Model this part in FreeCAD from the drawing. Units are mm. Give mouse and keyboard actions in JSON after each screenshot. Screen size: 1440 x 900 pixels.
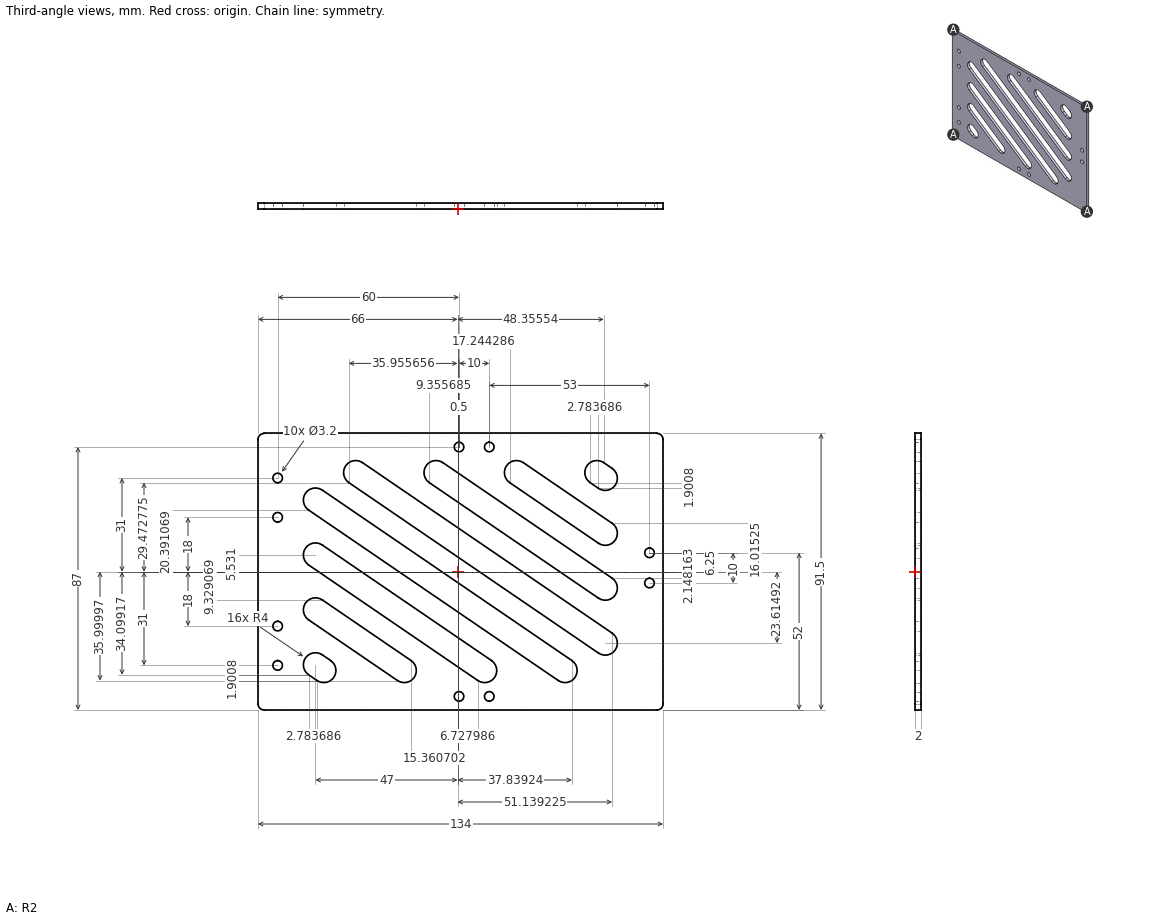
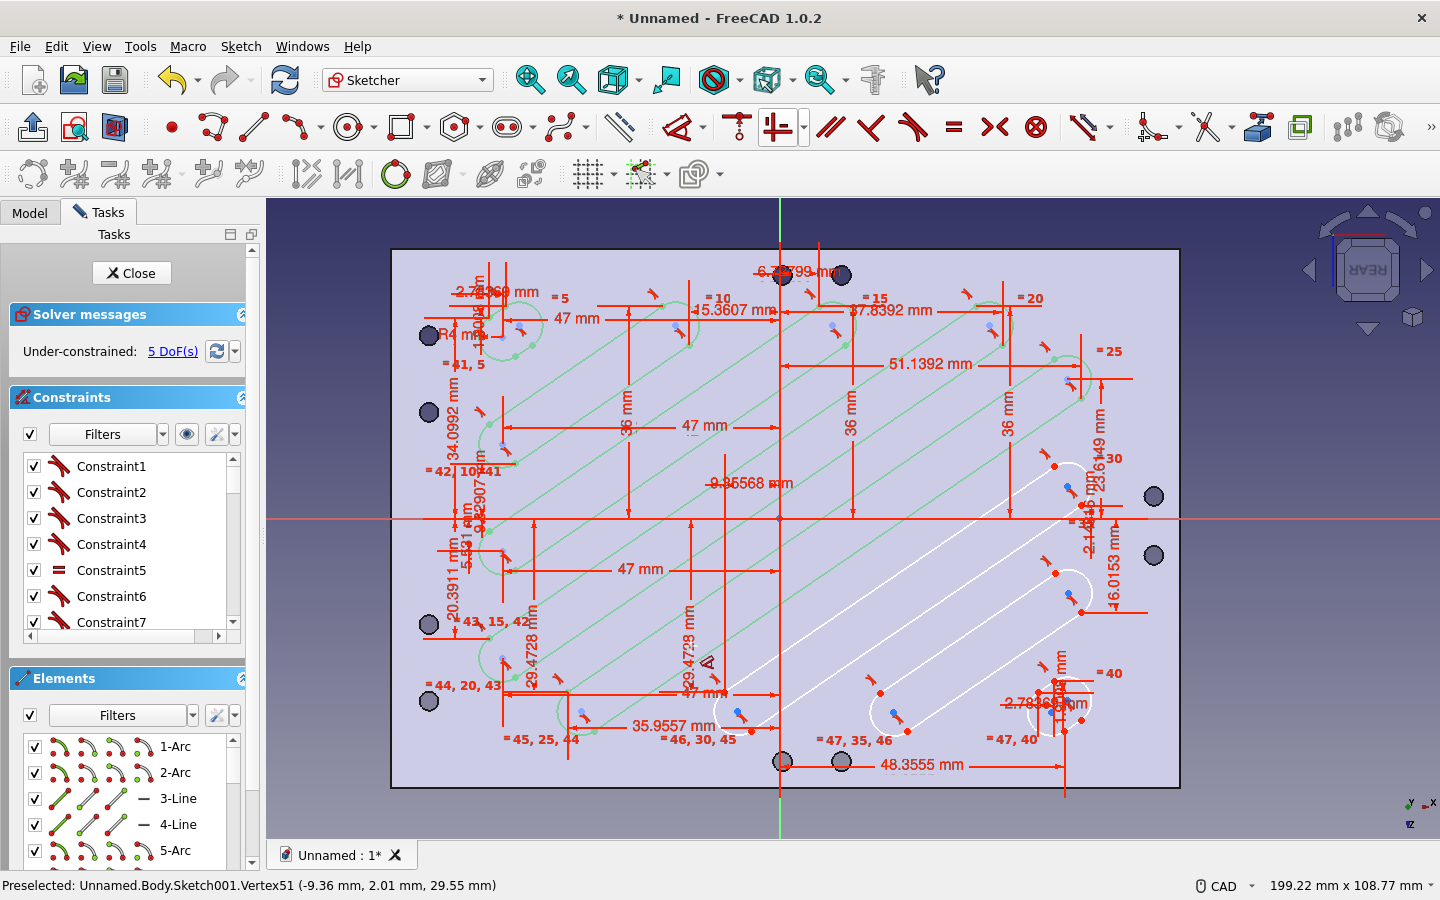
{"action": "left_click", "coordinate": [1081, 506]}
{"action": "left_click", "coordinate": [930, 472]}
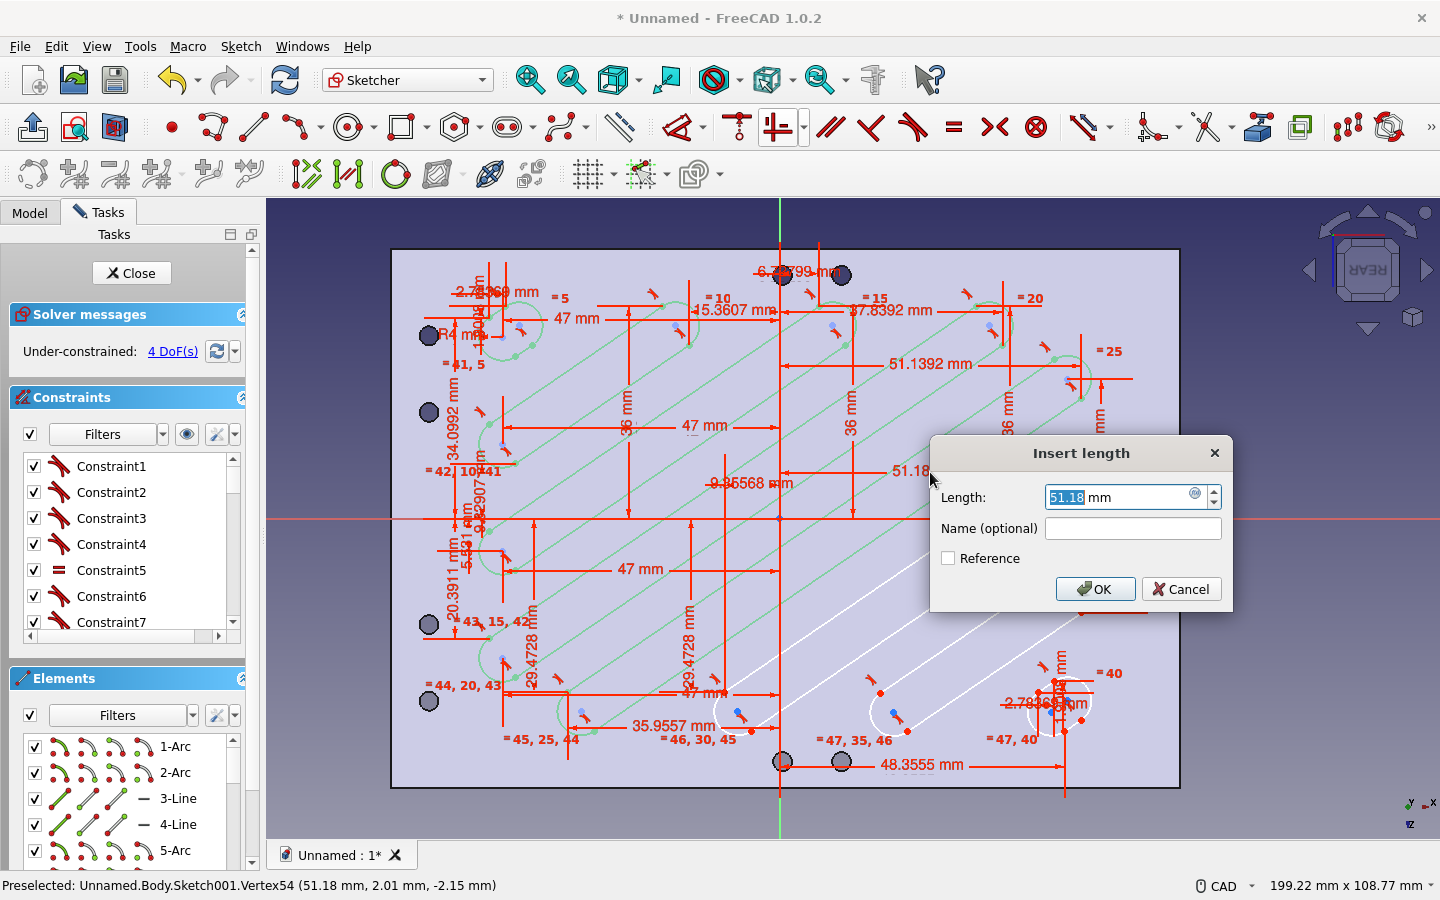
{"action": "type", "text": "51.139225"}
{"action": "key", "text": "Return"}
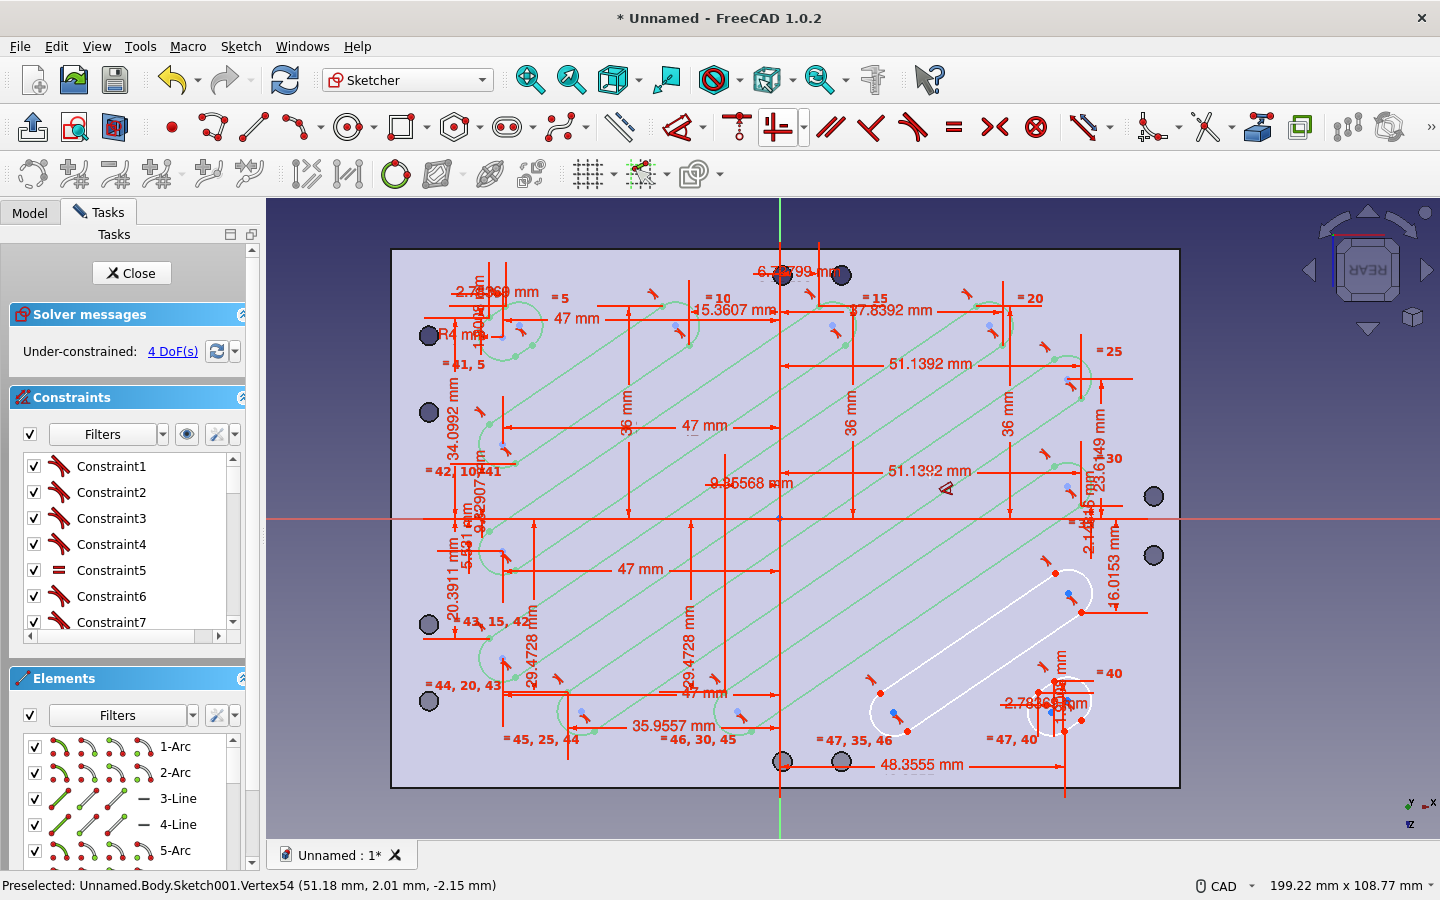
{"action": "left_click", "coordinate": [881, 693]}
{"action": "left_click", "coordinate": [830, 727]}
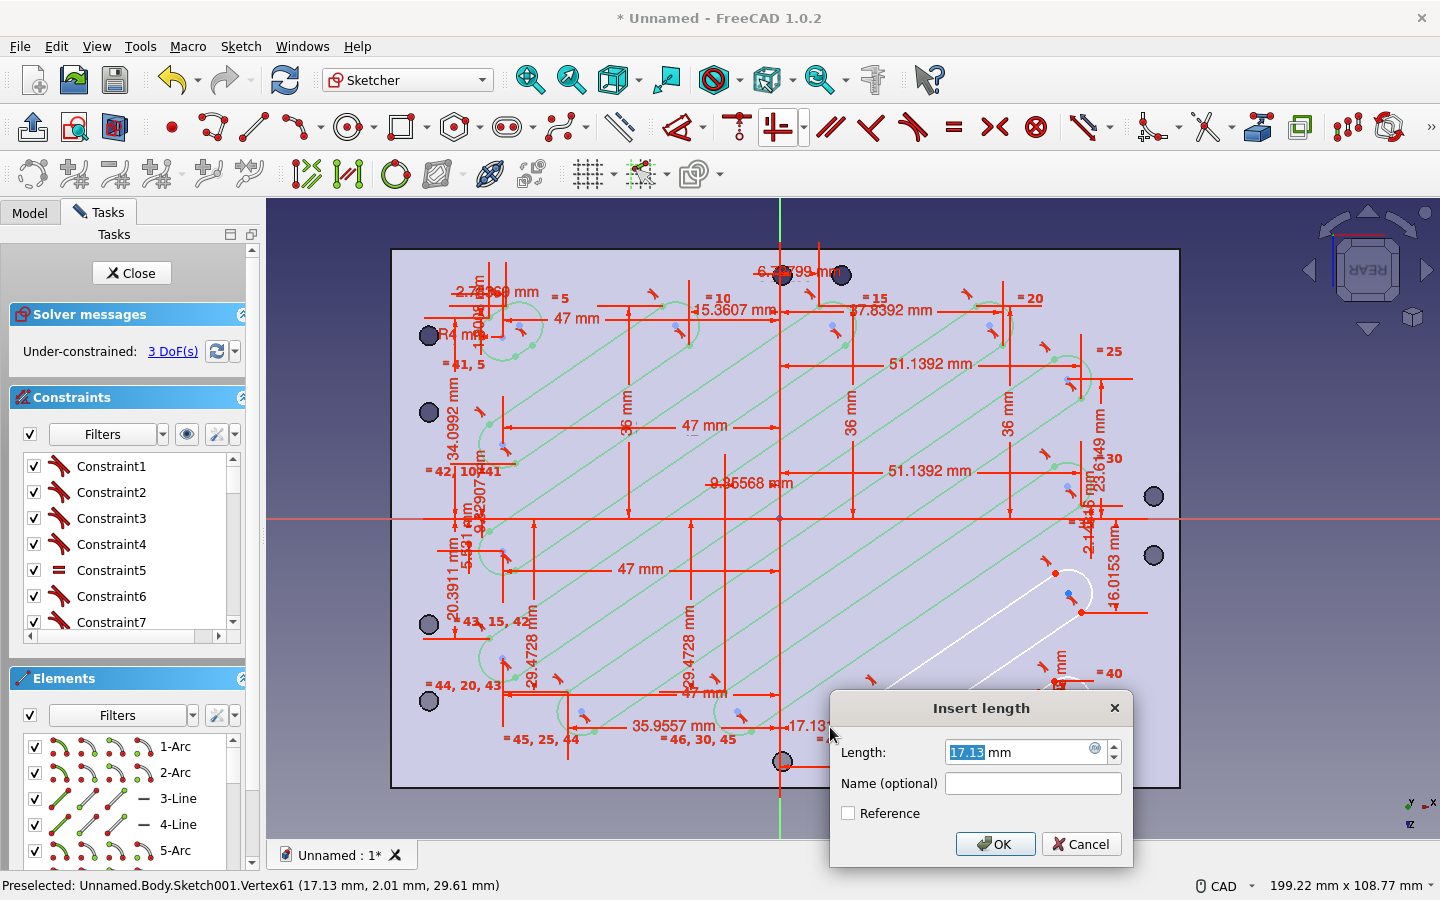
{"action": "type", "text": "17.244286"}
{"action": "key", "text": "Return"}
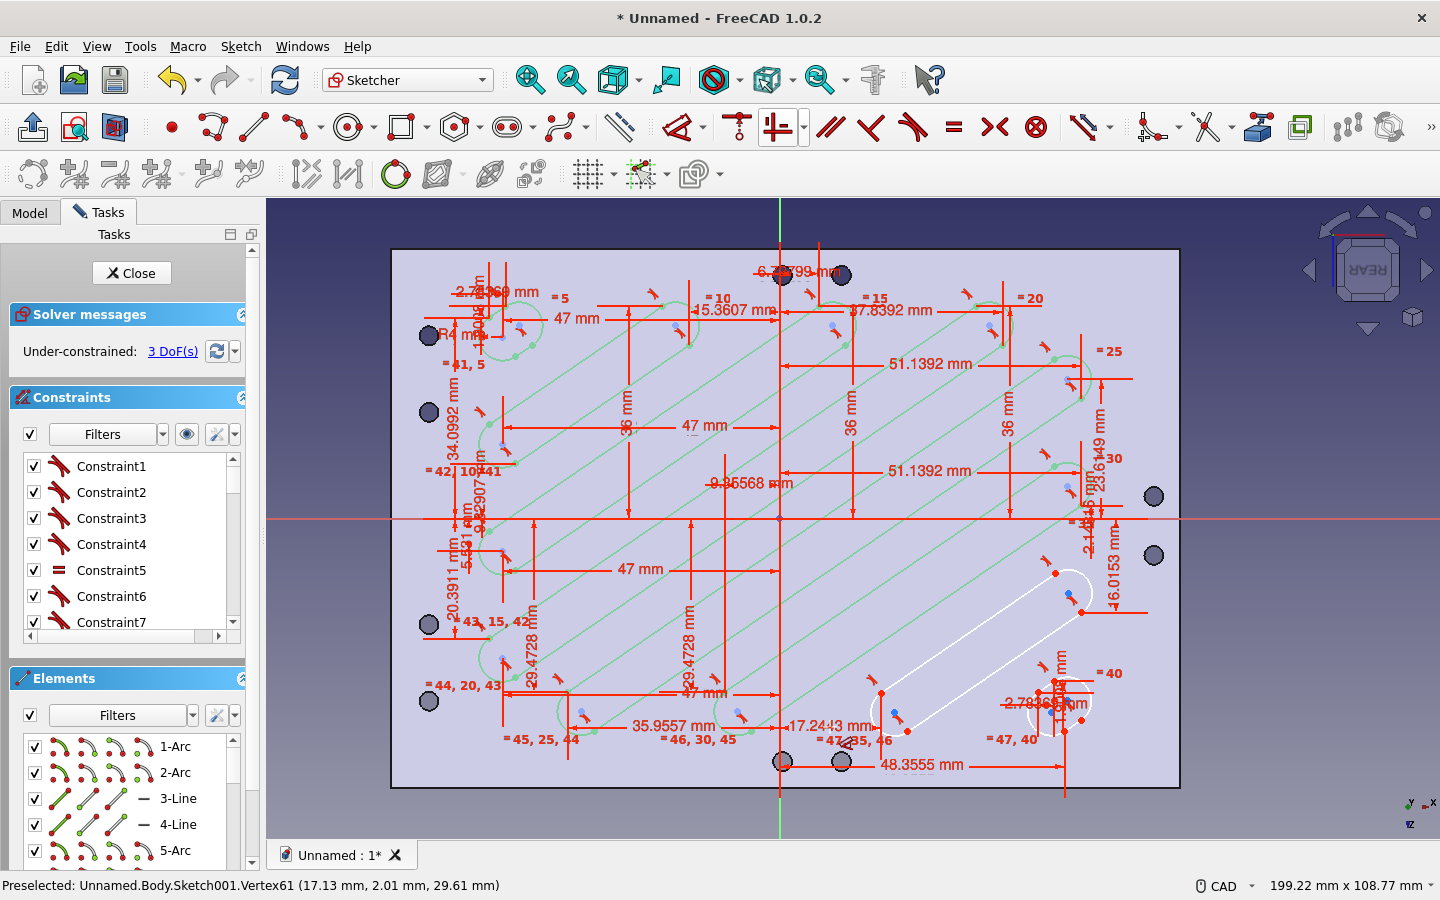
{"action": "left_click", "coordinate": [881, 693]}
{"action": "left_click", "coordinate": [915, 646]}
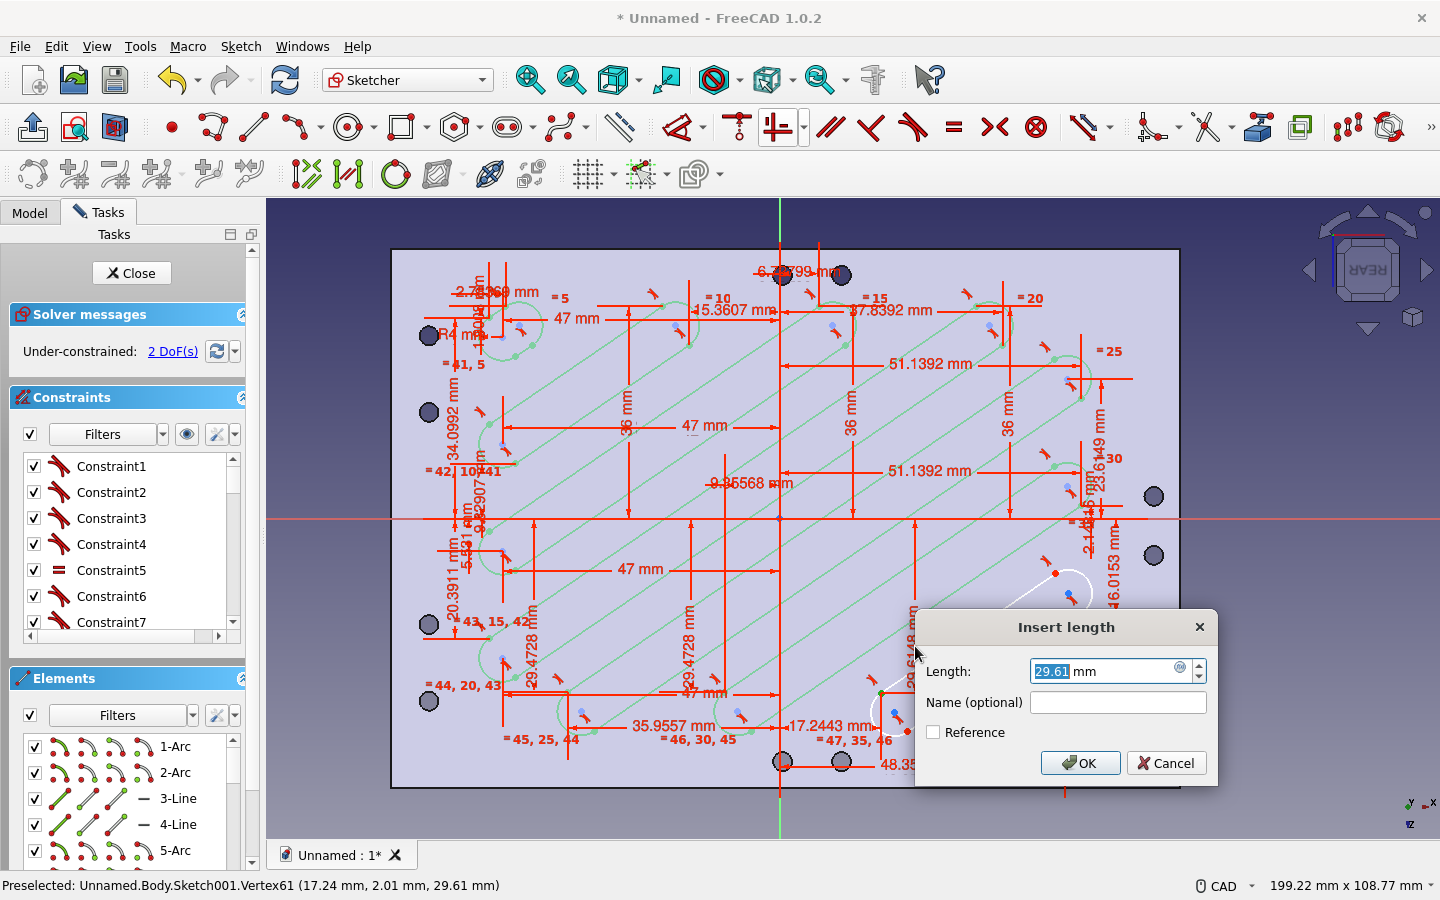
{"action": "type", "text": "29.472775"}
{"action": "key", "text": "Return"}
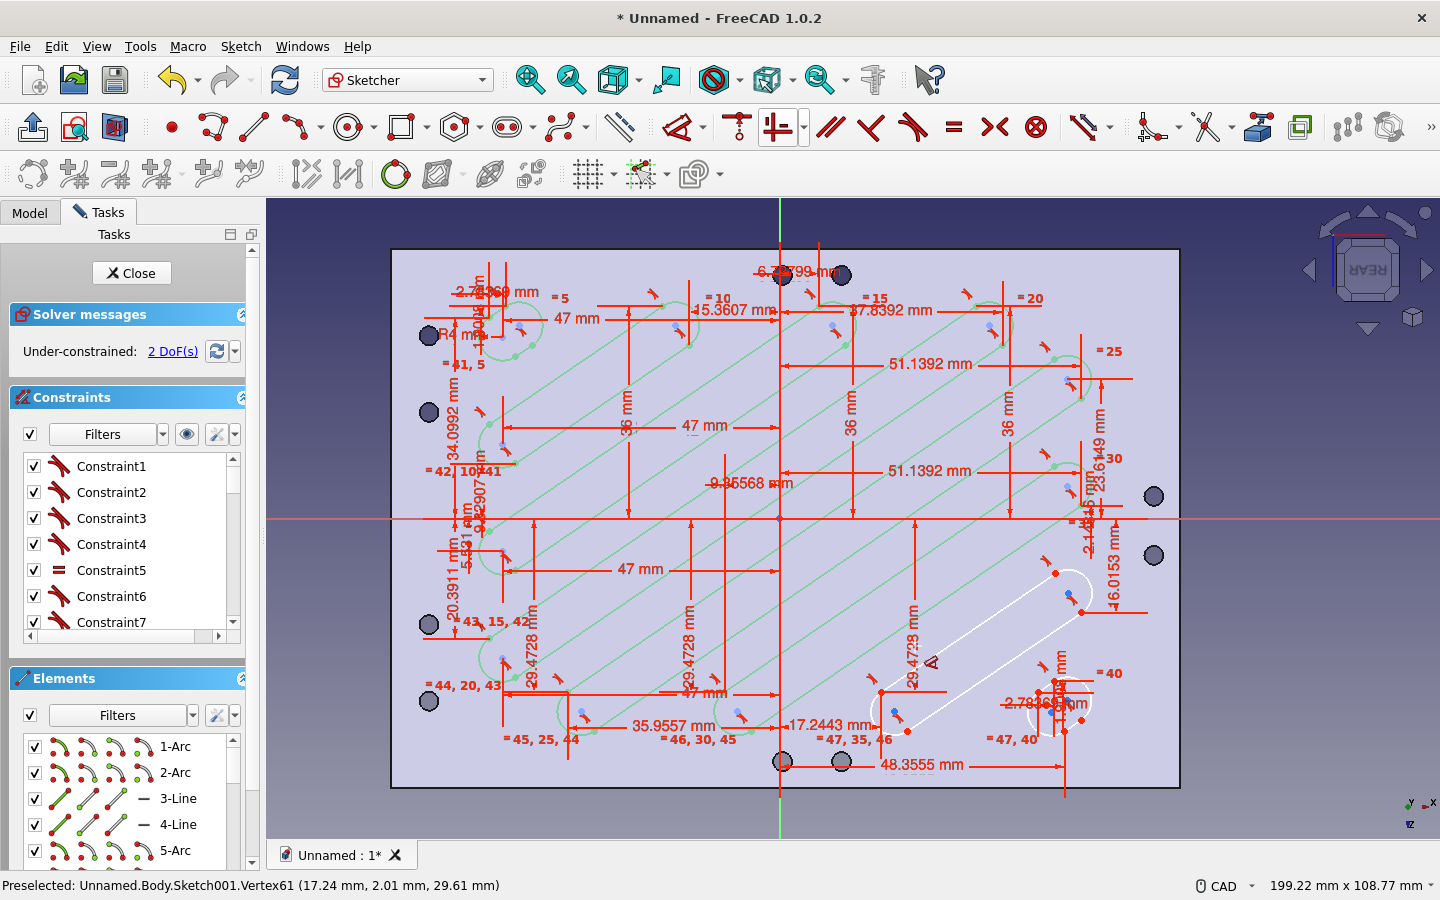
{"action": "left_click", "coordinate": [1082, 613]}
{"action": "left_click", "coordinate": [1000, 647]}